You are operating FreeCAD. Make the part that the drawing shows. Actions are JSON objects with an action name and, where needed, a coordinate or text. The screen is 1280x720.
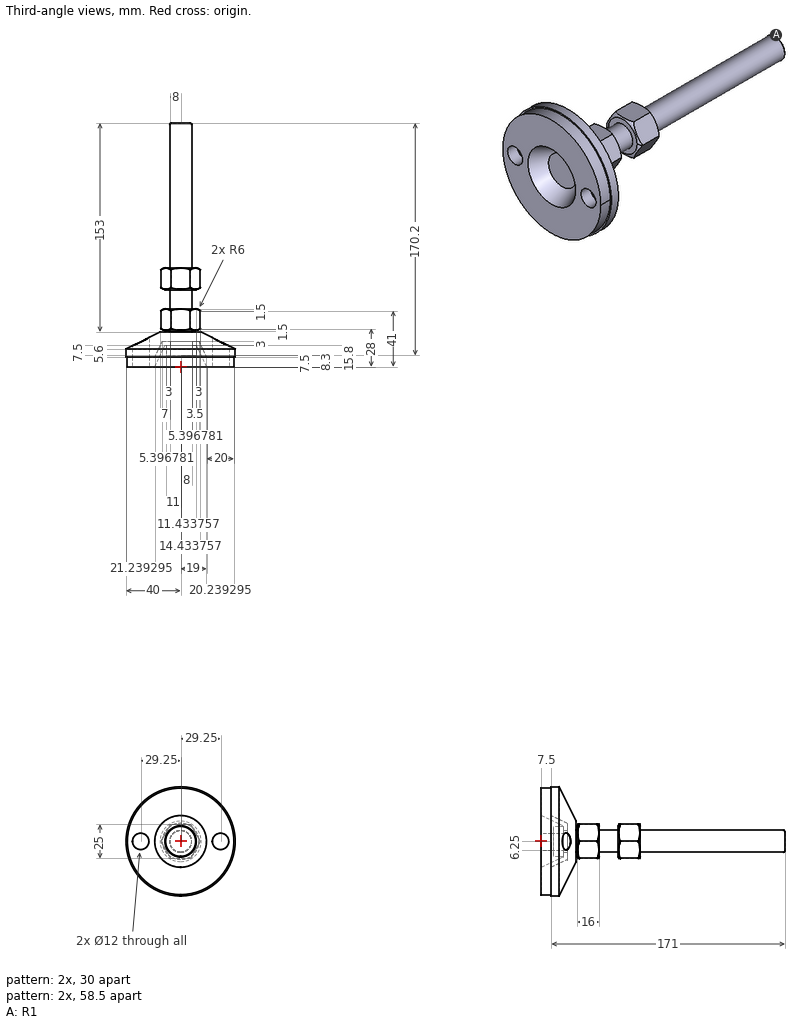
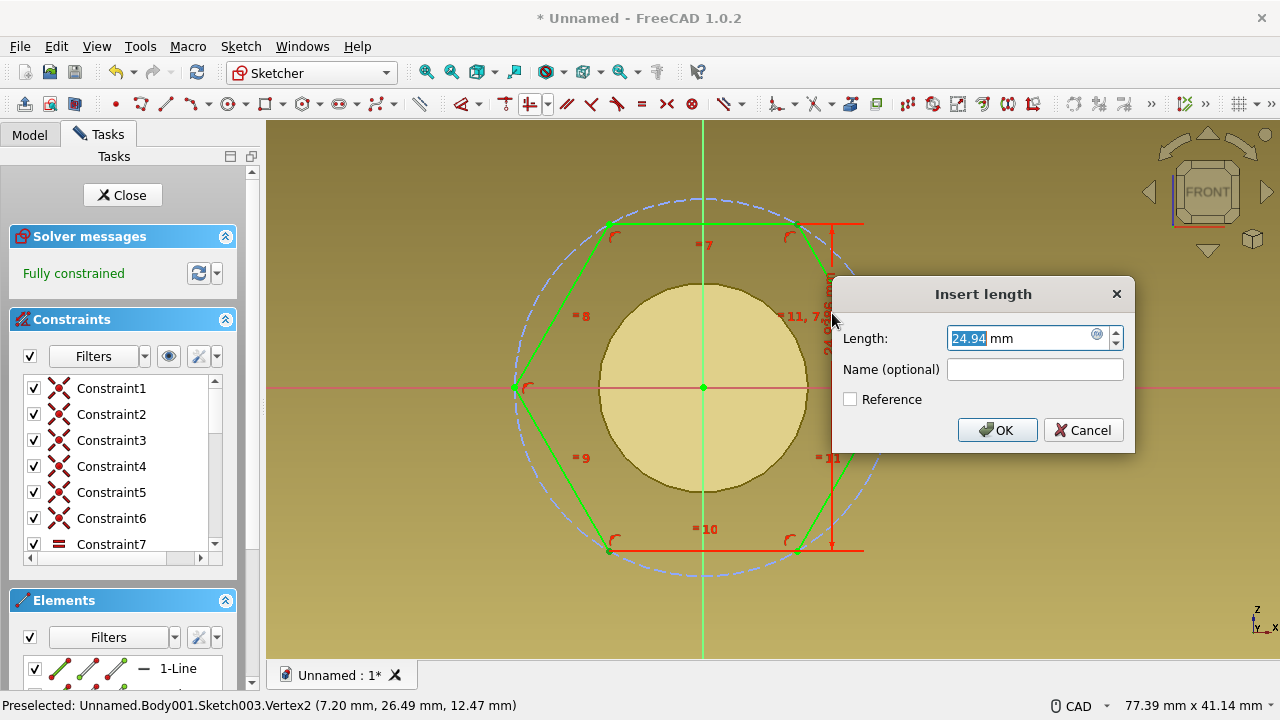
{"action": "type", "text": "25"}
{"action": "key", "text": "Return"}
{"action": "key", "text": "Escape"}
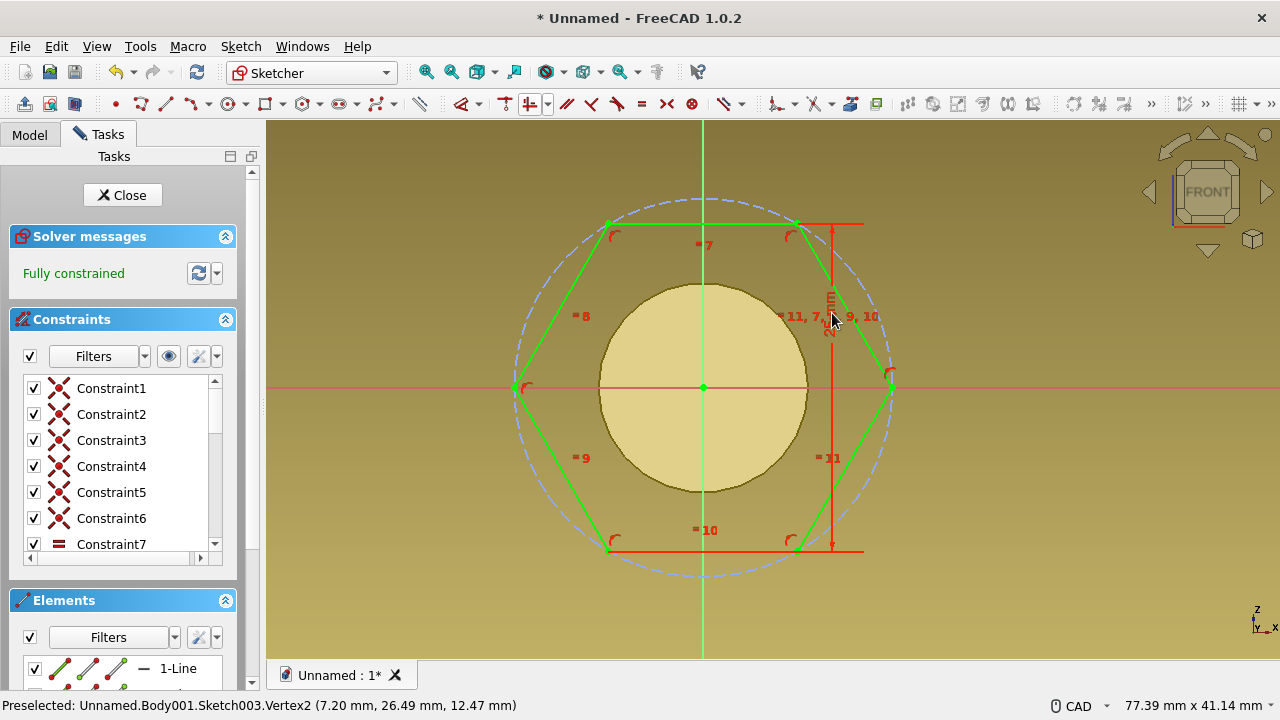
{"action": "left_click", "coordinate": [123, 195]}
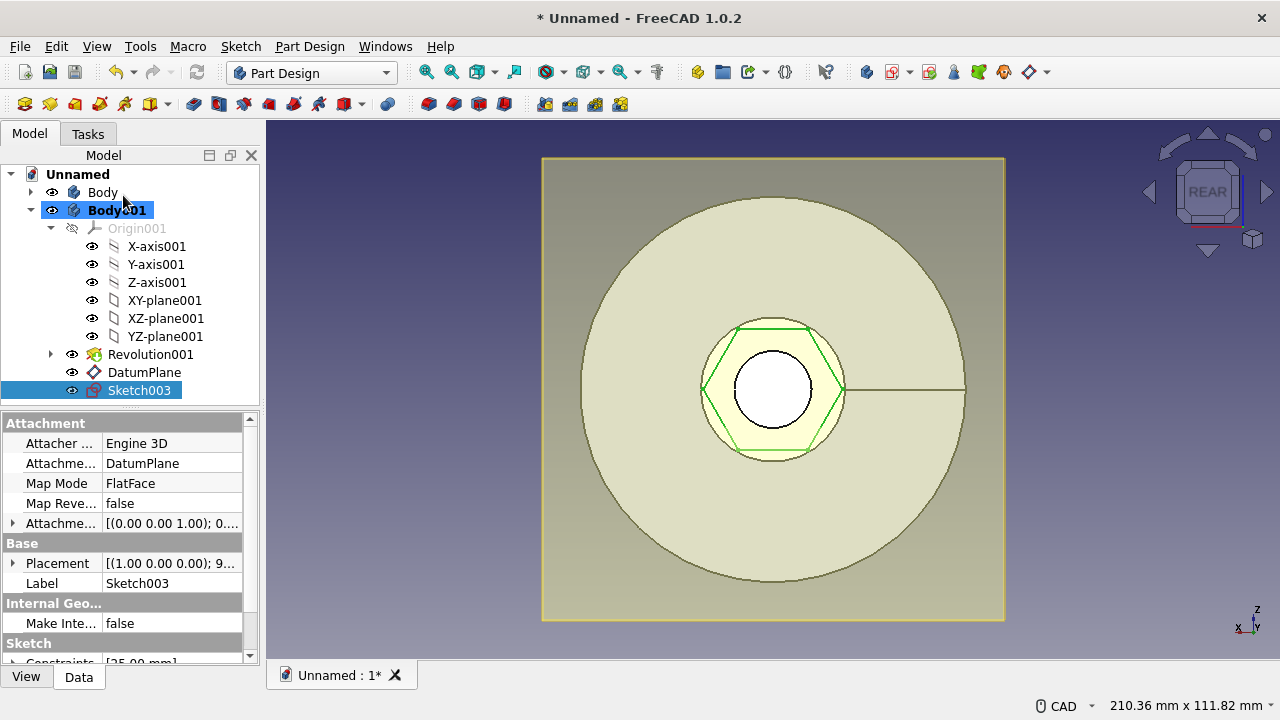
{"action": "left_click", "coordinate": [25, 104]}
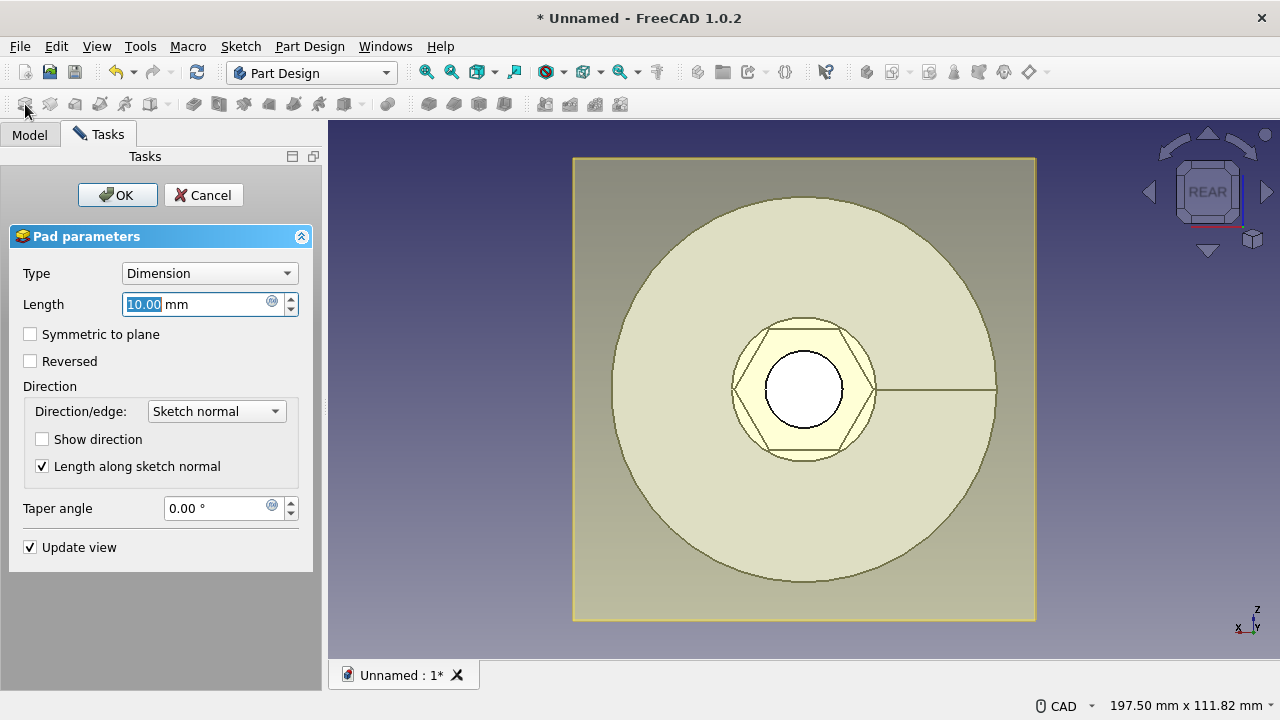
{"action": "type", "text": "16"}
{"action": "key", "text": "Tab"}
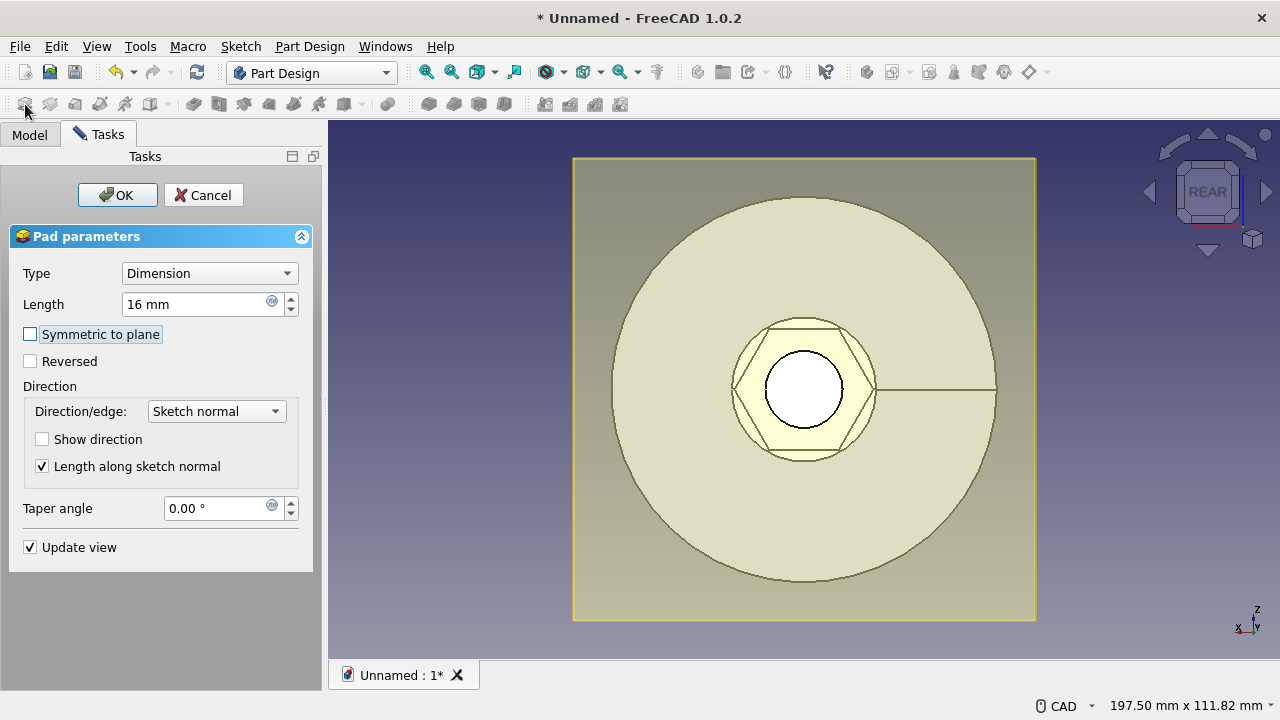
{"action": "left_click", "coordinate": [31, 361]}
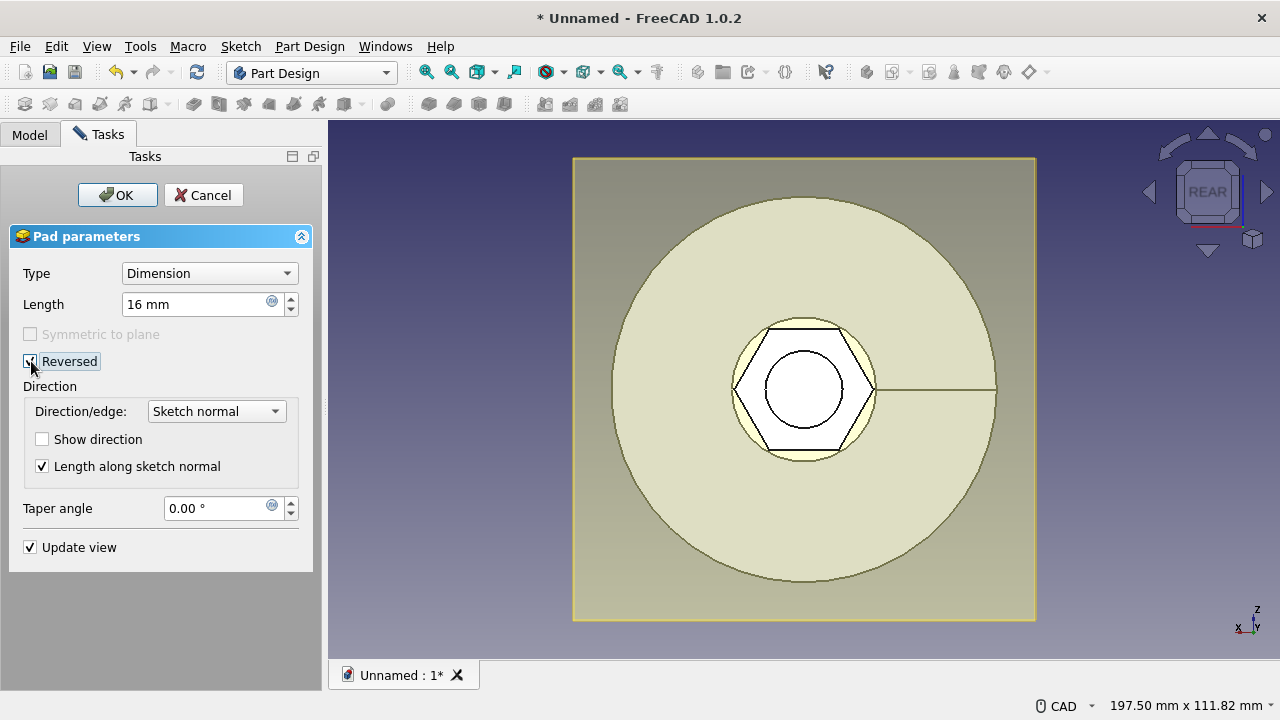
{"action": "left_click", "coordinate": [118, 195]}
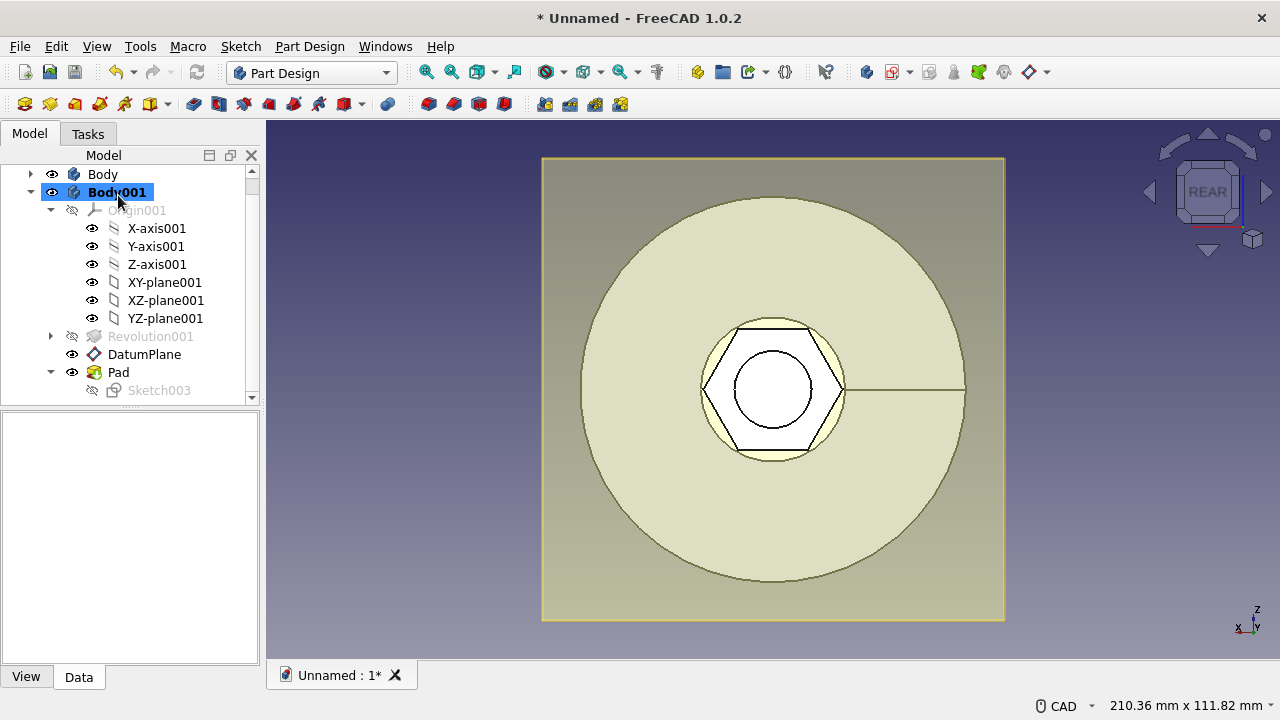
{"action": "left_click", "coordinate": [117, 354]}
{"action": "key", "text": "space"}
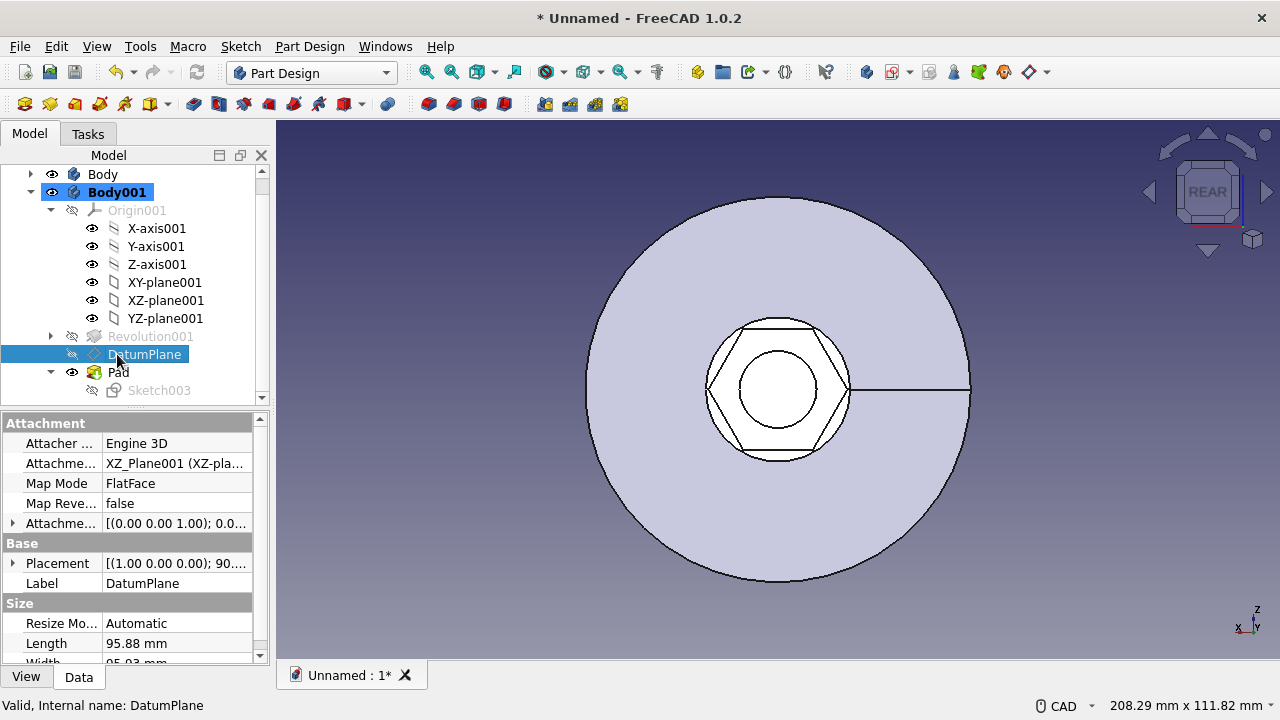
{"action": "left_click", "coordinate": [316, 619]}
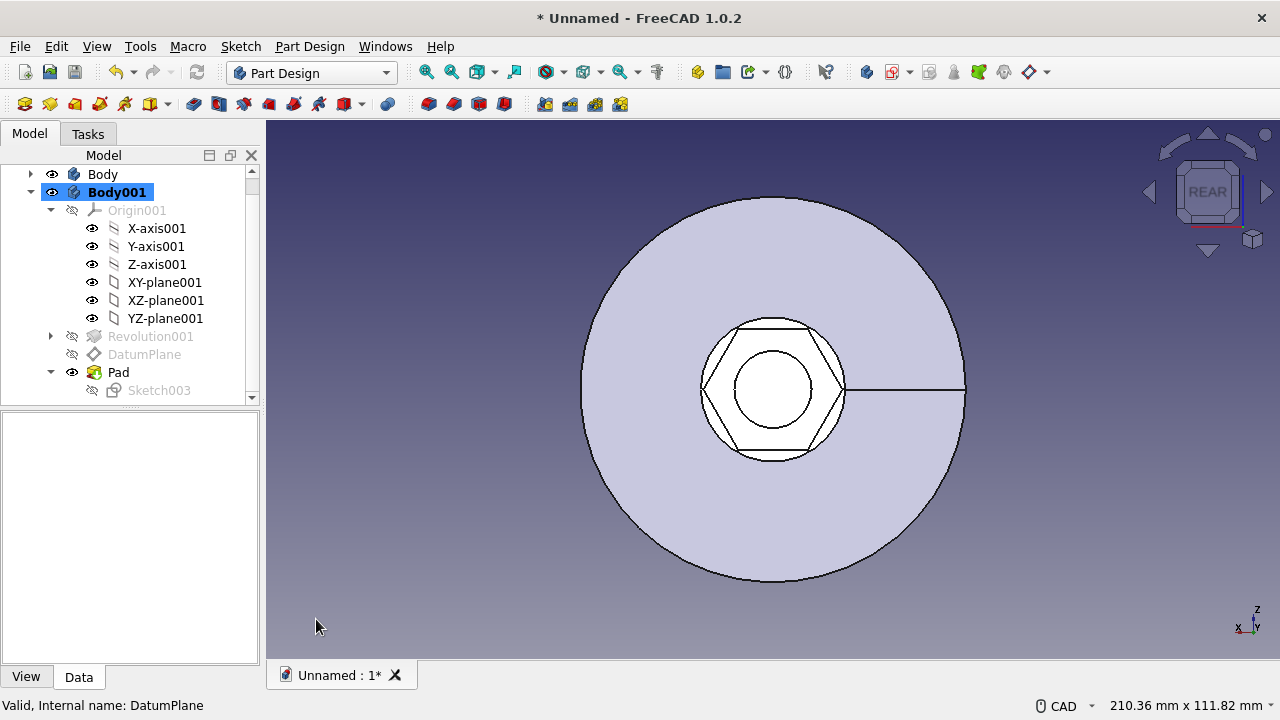
{"action": "left_click", "coordinate": [892, 72]}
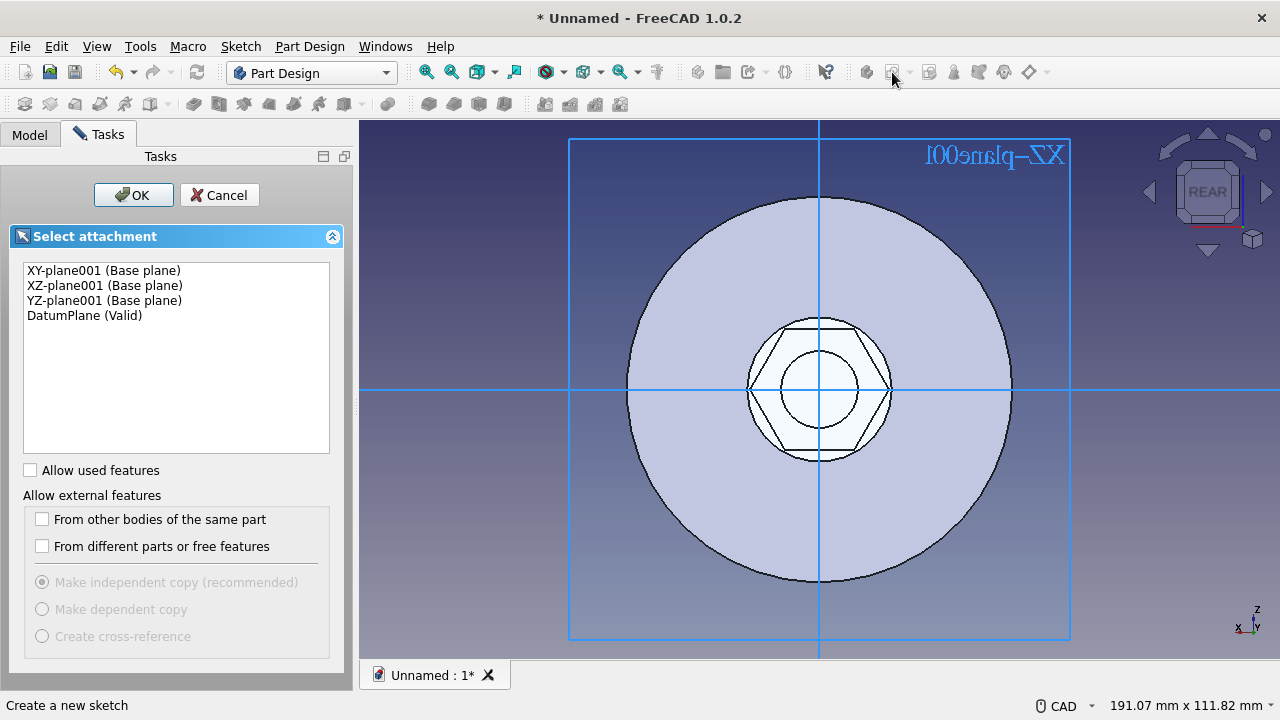
{"action": "left_click", "coordinate": [84, 270]}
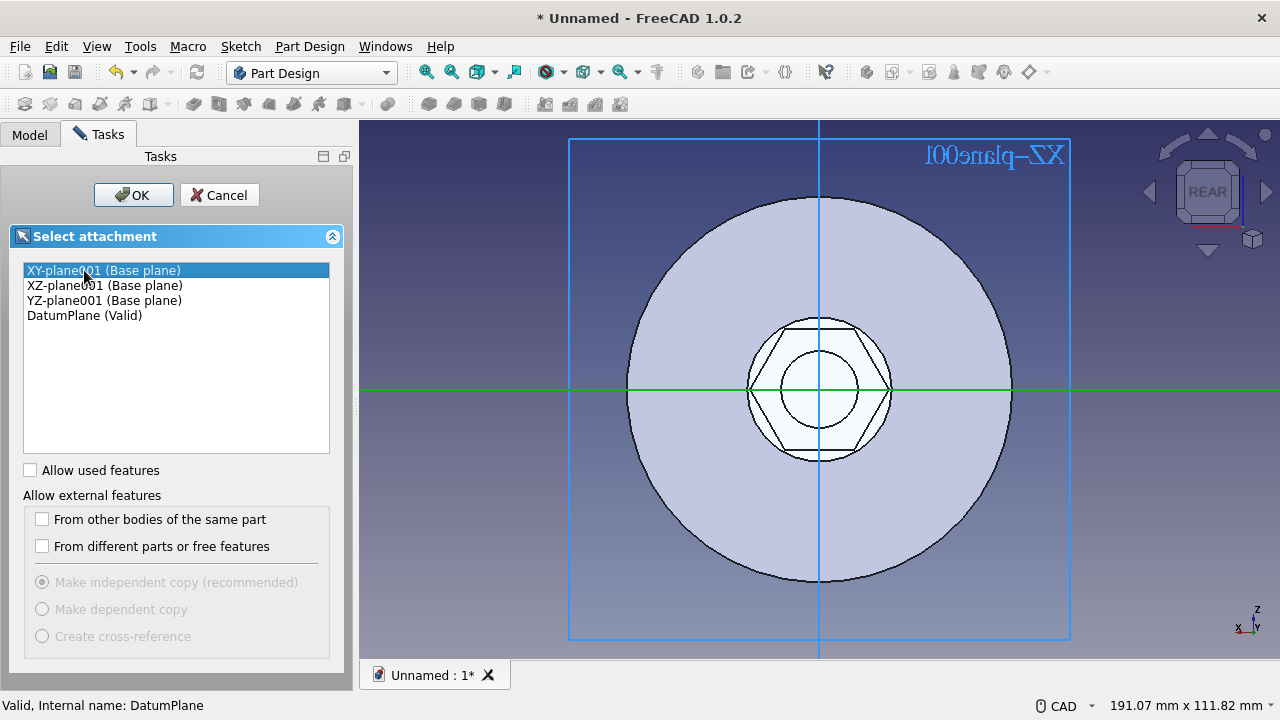
{"action": "left_click", "coordinate": [134, 195]}